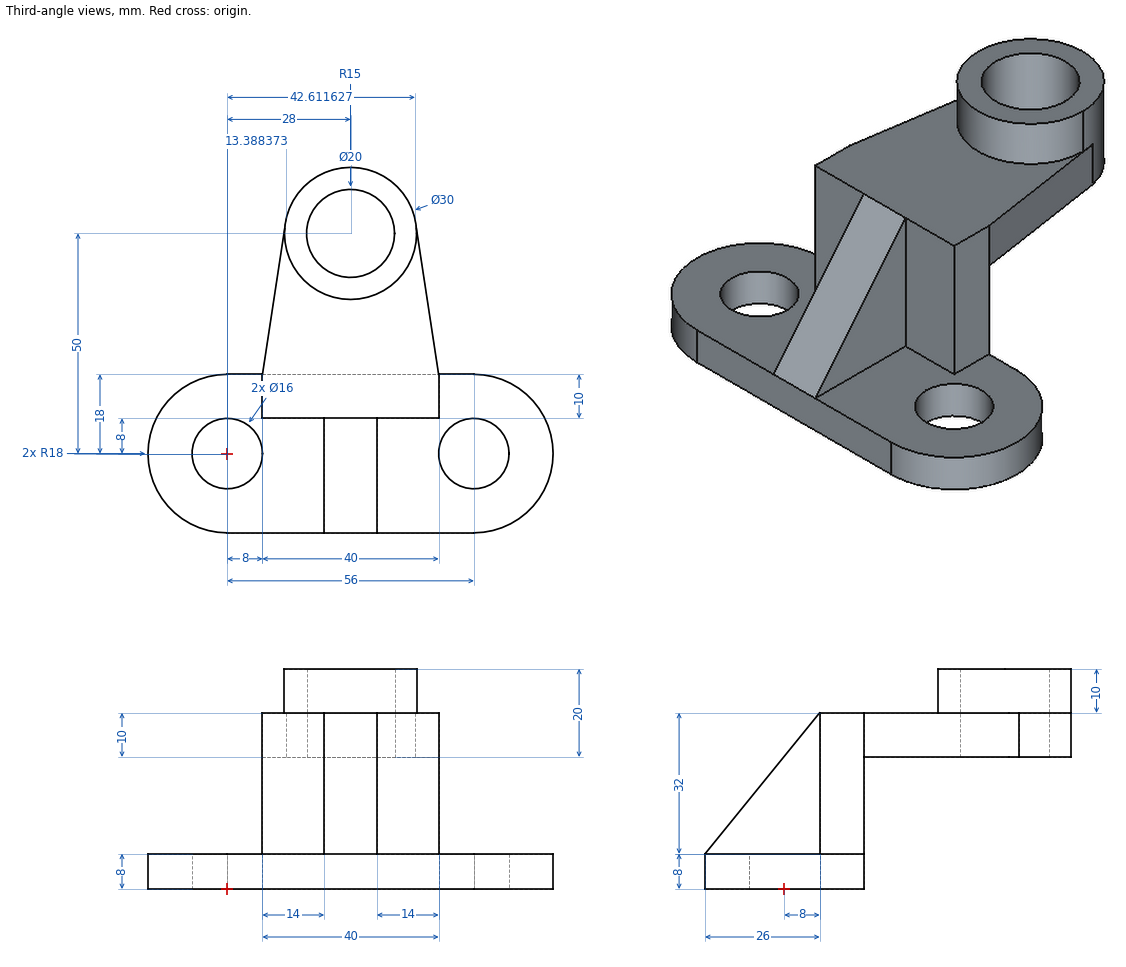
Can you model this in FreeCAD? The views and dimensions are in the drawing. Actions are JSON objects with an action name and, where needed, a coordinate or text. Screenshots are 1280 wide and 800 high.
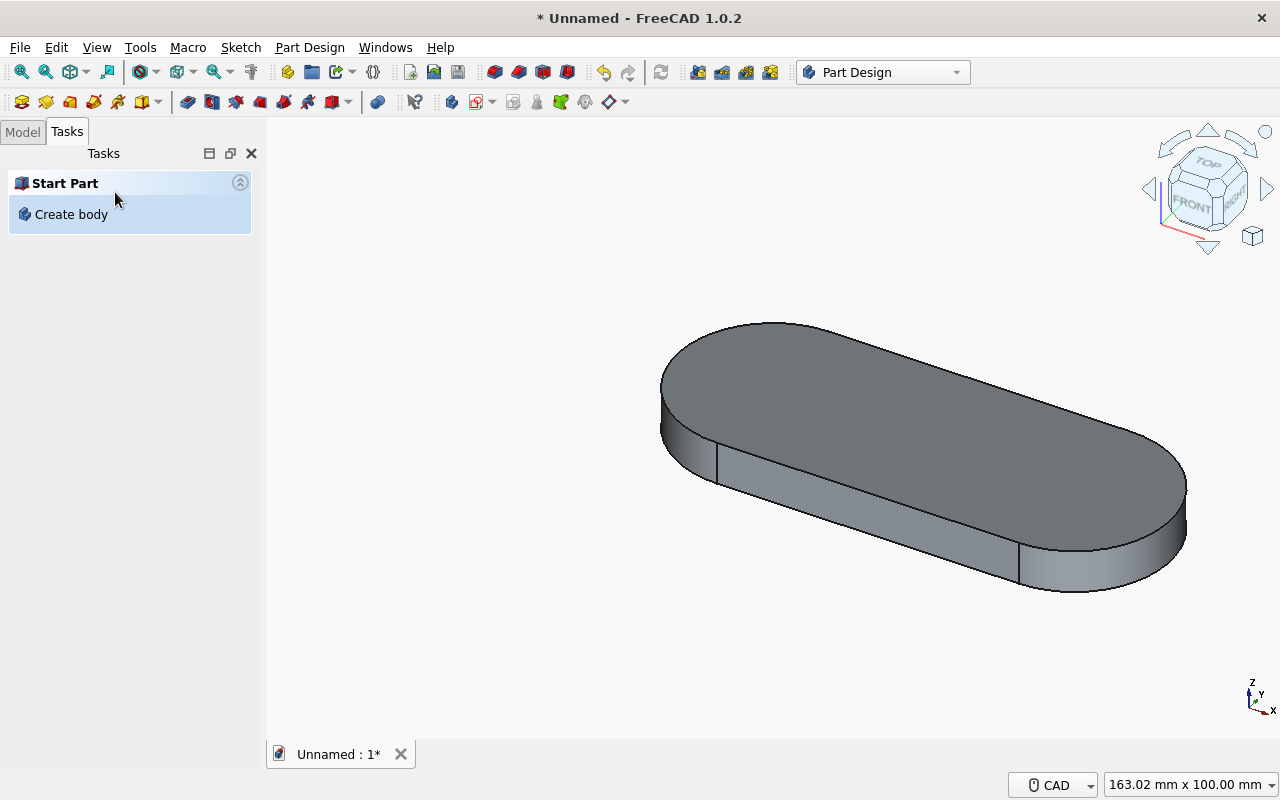
{"action": "left_click", "coordinate": [1065, 483]}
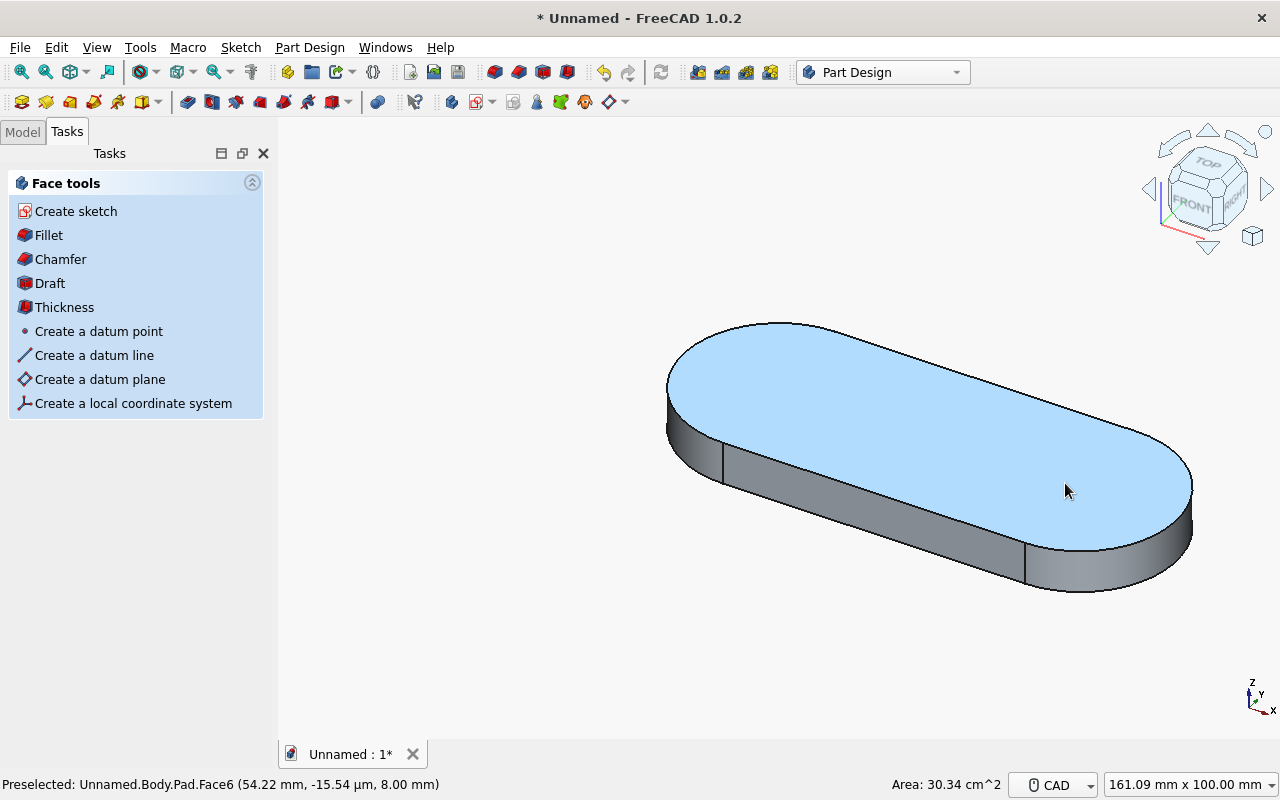
{"action": "left_click", "coordinate": [476, 102]}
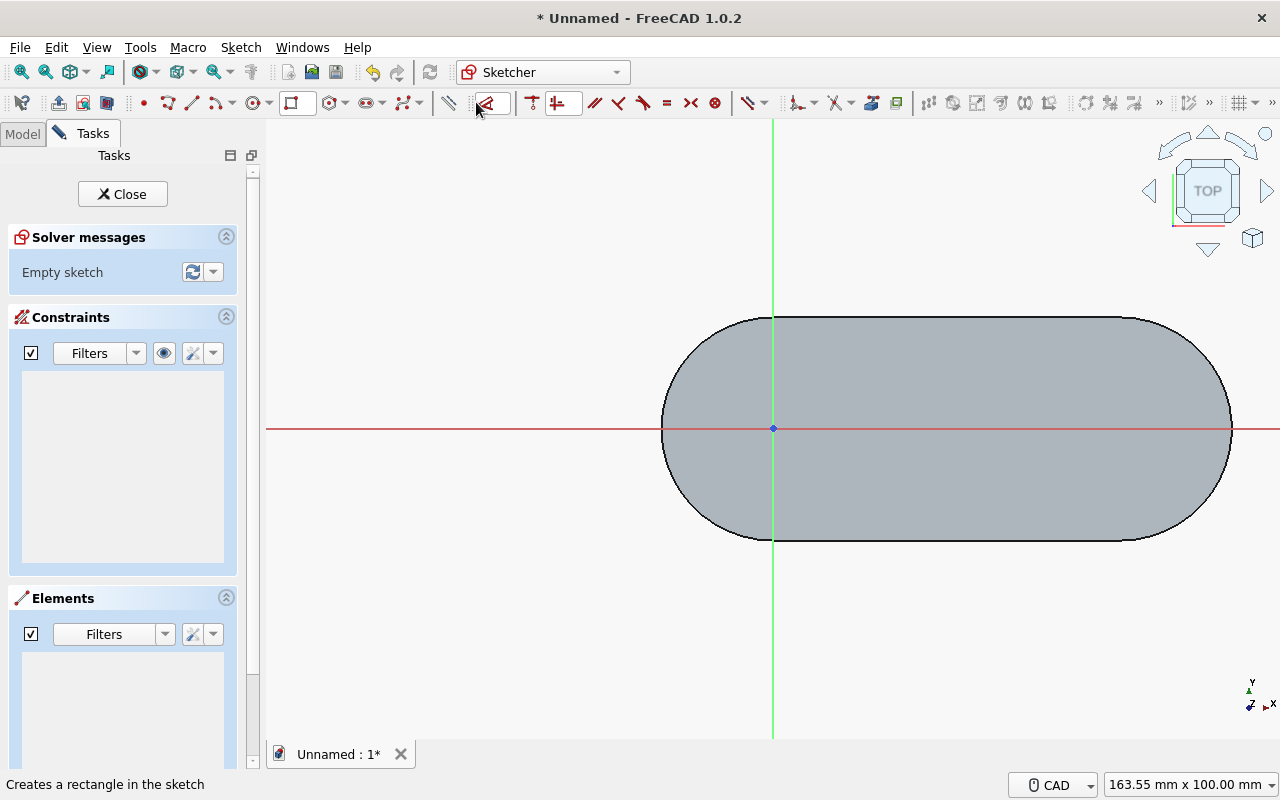
{"action": "scroll", "coordinate": [294, 429], "scroll_direction": "down", "scroll_amount": 1}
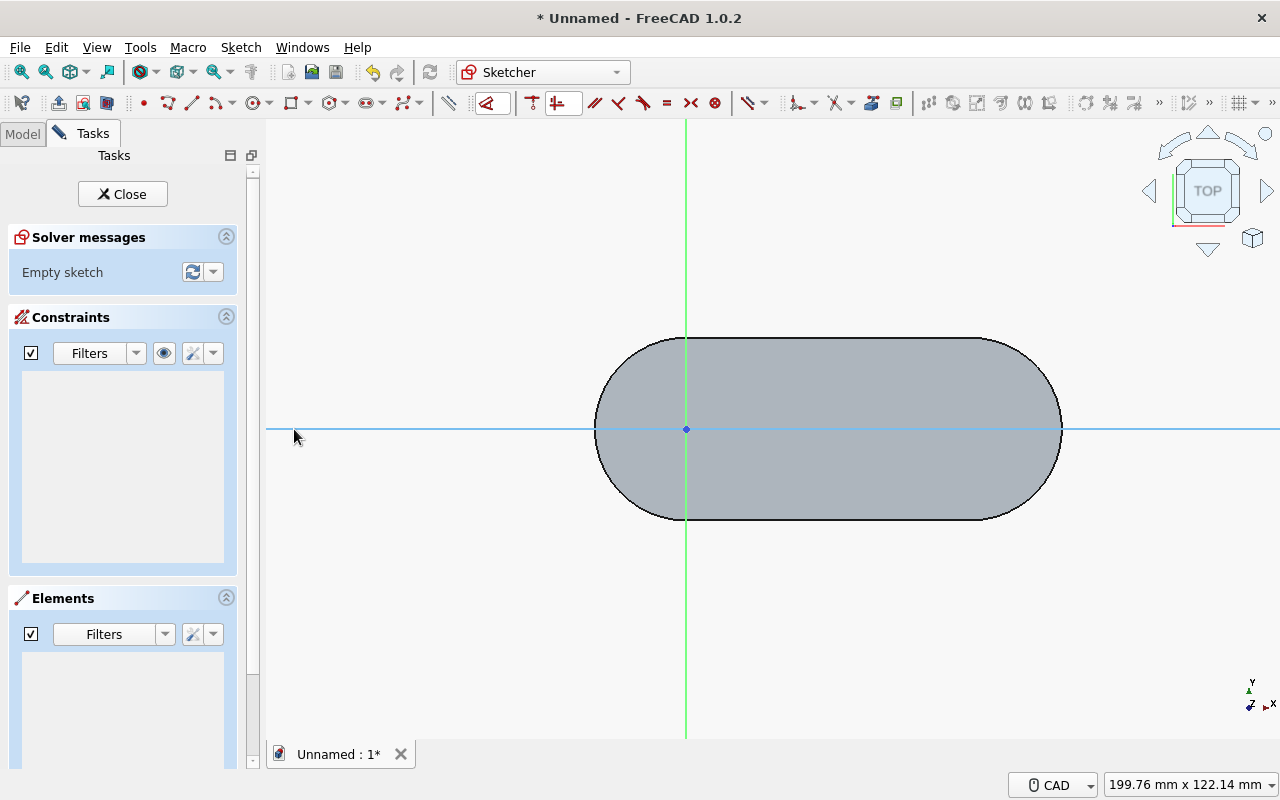
{"action": "scroll", "coordinate": [1080, 429], "scroll_direction": "up", "scroll_amount": 2}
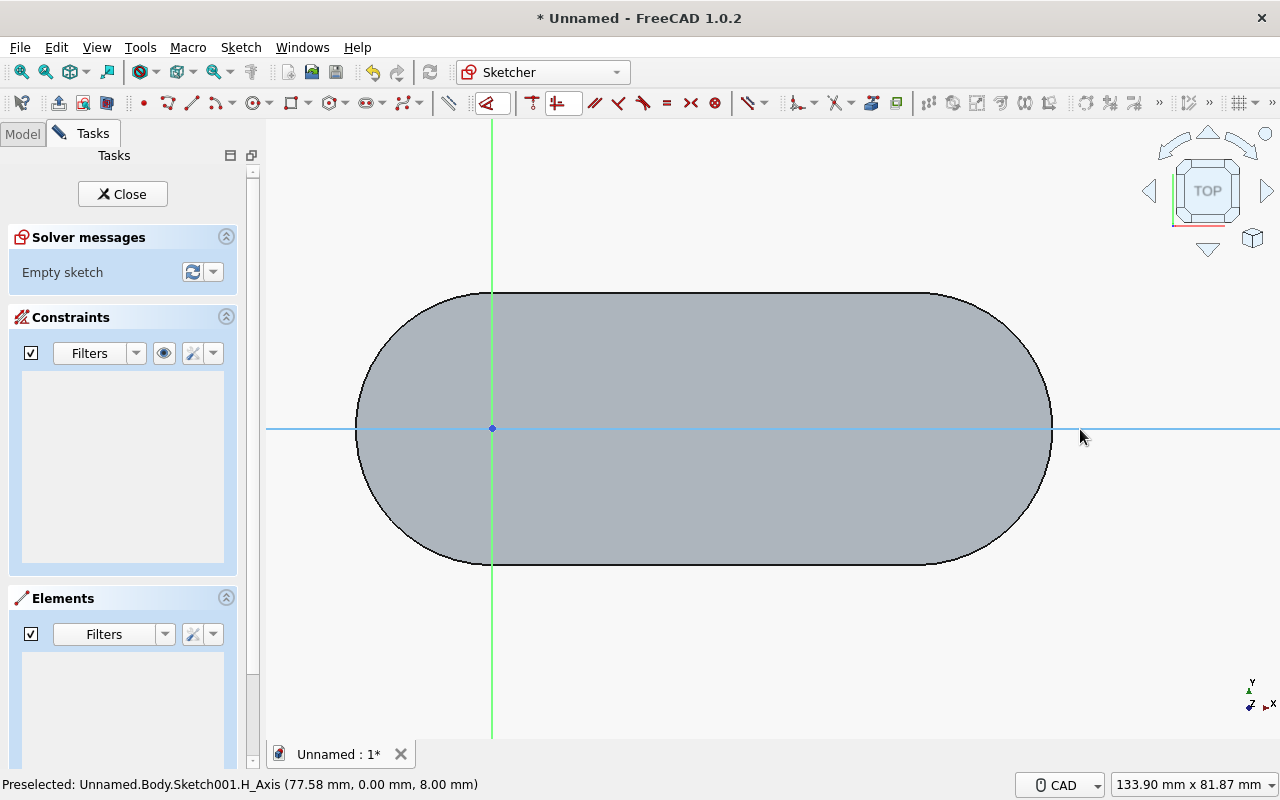
{"action": "left_click", "coordinate": [254, 104]}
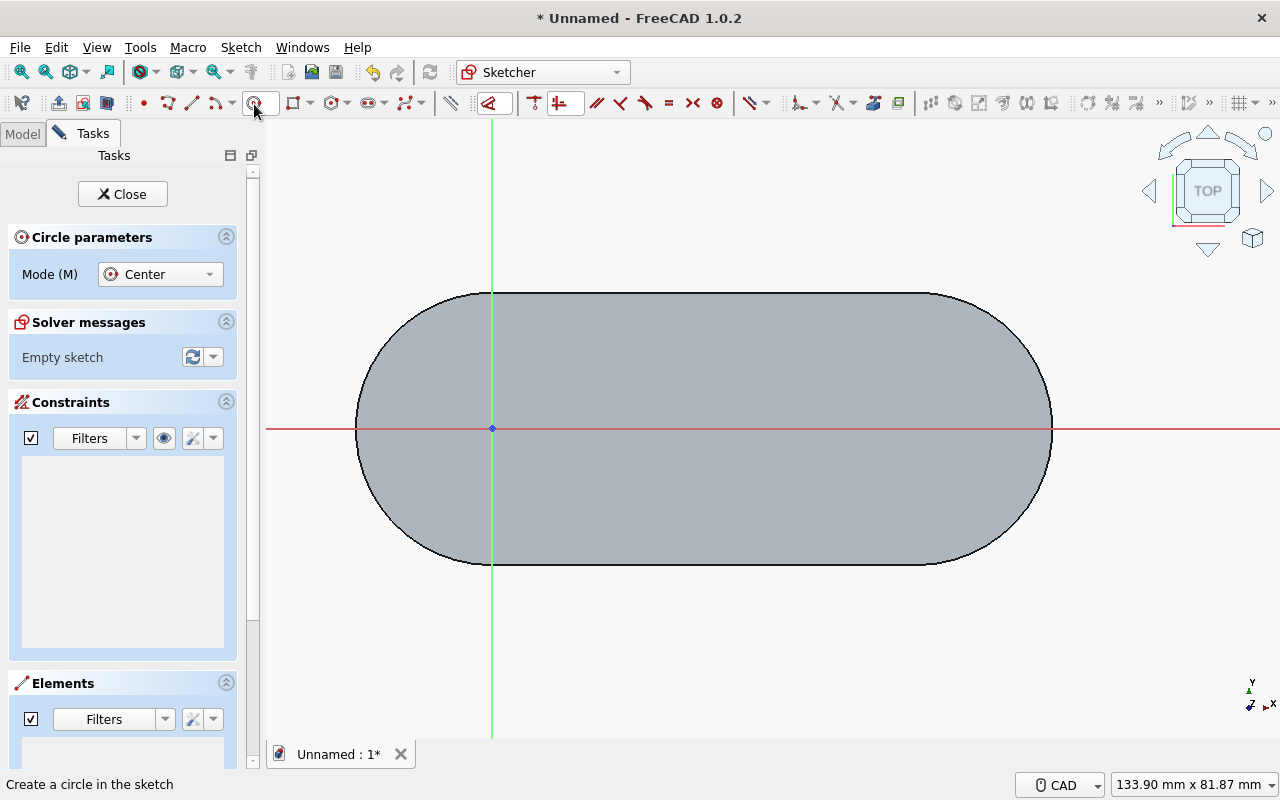
{"action": "left_click", "coordinate": [492, 429]}
{"action": "mouse_move", "coordinate": [535, 386]}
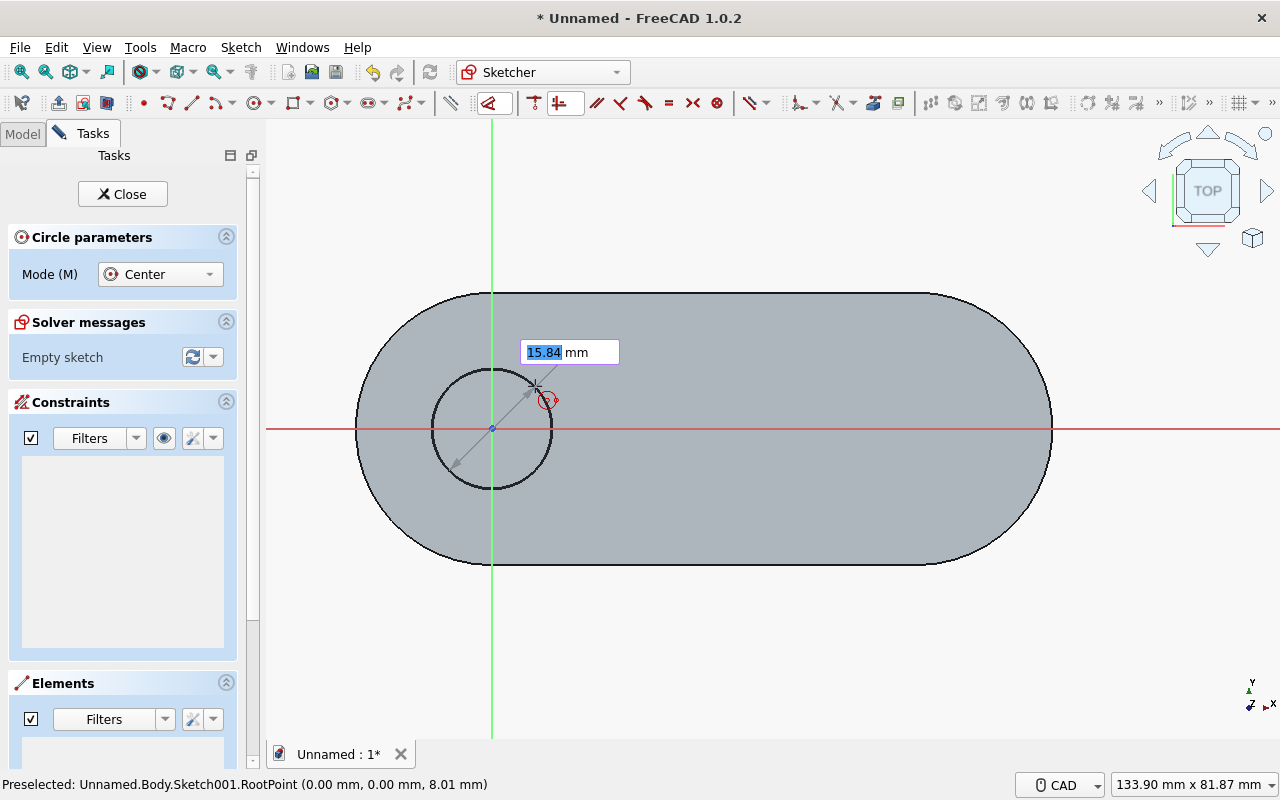
{"action": "type", "text": "16"}
{"action": "key", "text": "Return"}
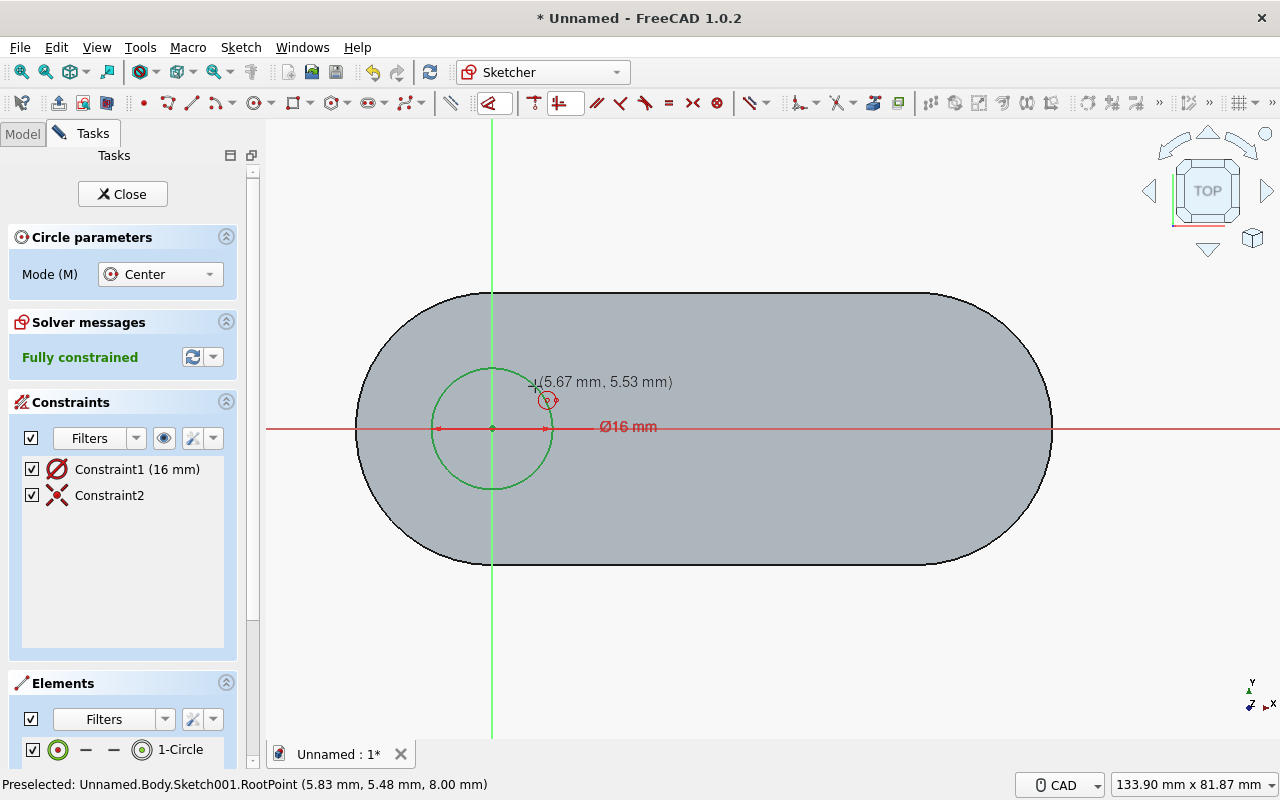
{"action": "left_click", "coordinate": [916, 429]}
{"action": "mouse_move", "coordinate": [959, 386]}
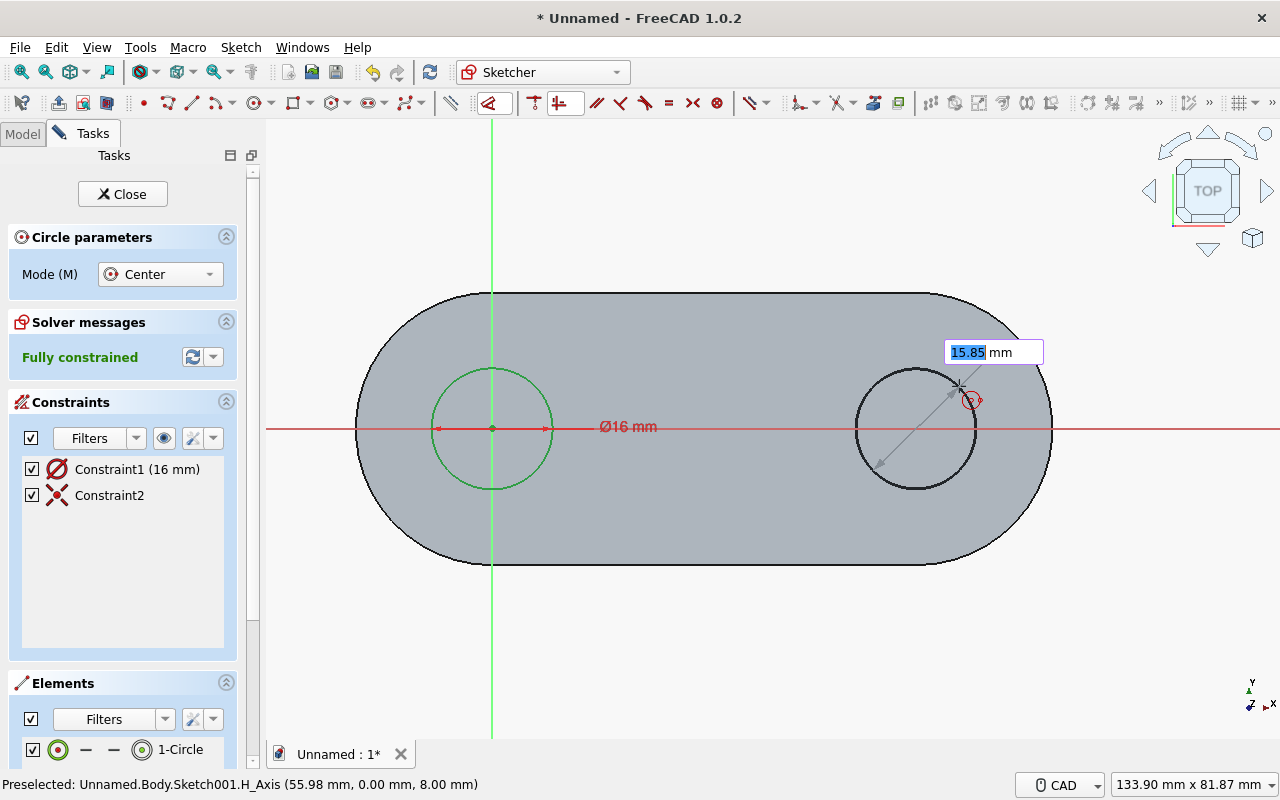
{"action": "type", "text": "16"}
{"action": "key", "text": "Return"}
{"action": "key", "text": "Escape"}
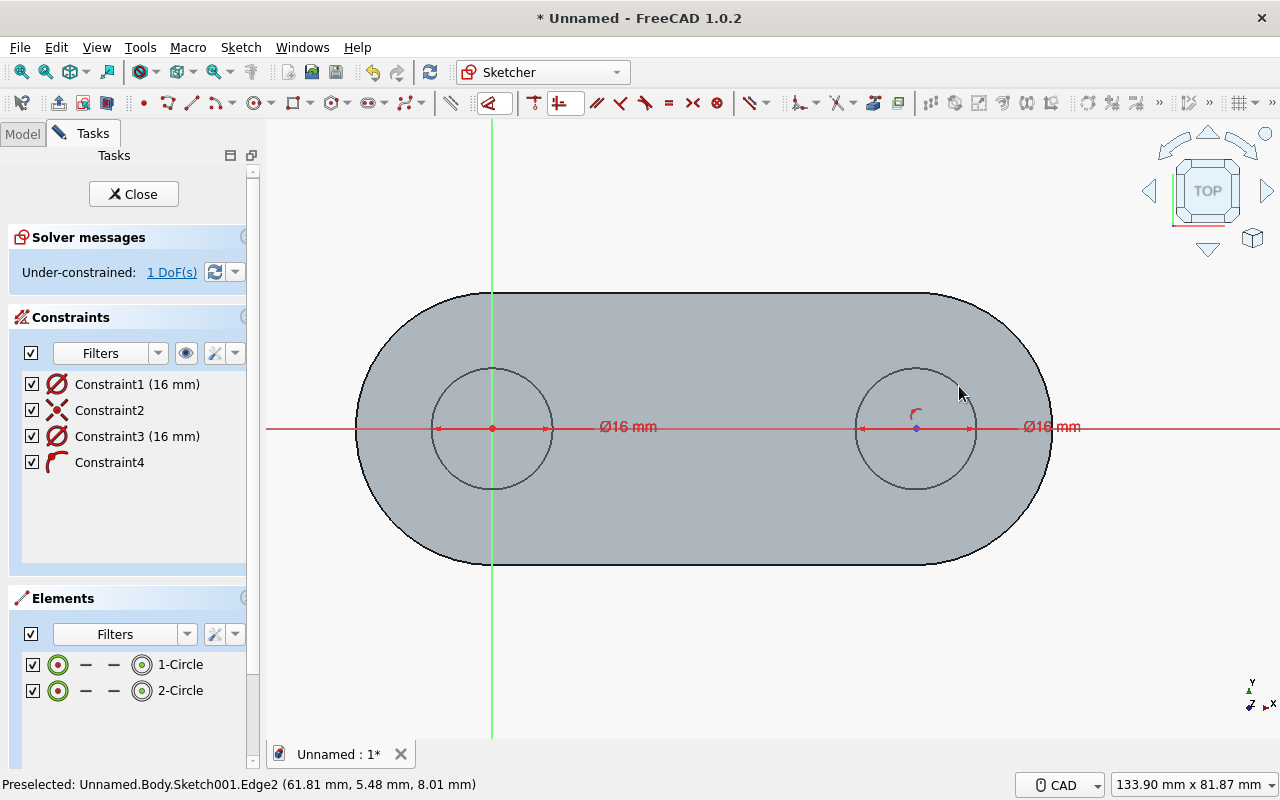
{"action": "left_click", "coordinate": [916, 429]}